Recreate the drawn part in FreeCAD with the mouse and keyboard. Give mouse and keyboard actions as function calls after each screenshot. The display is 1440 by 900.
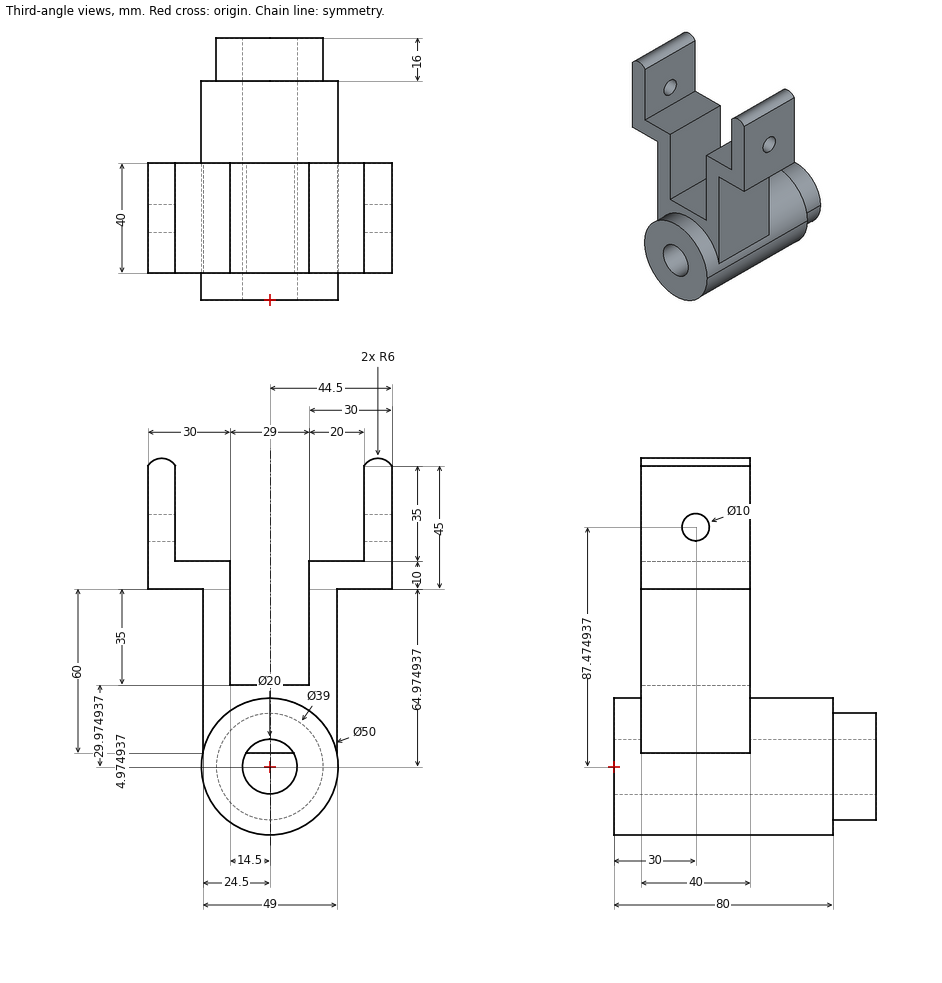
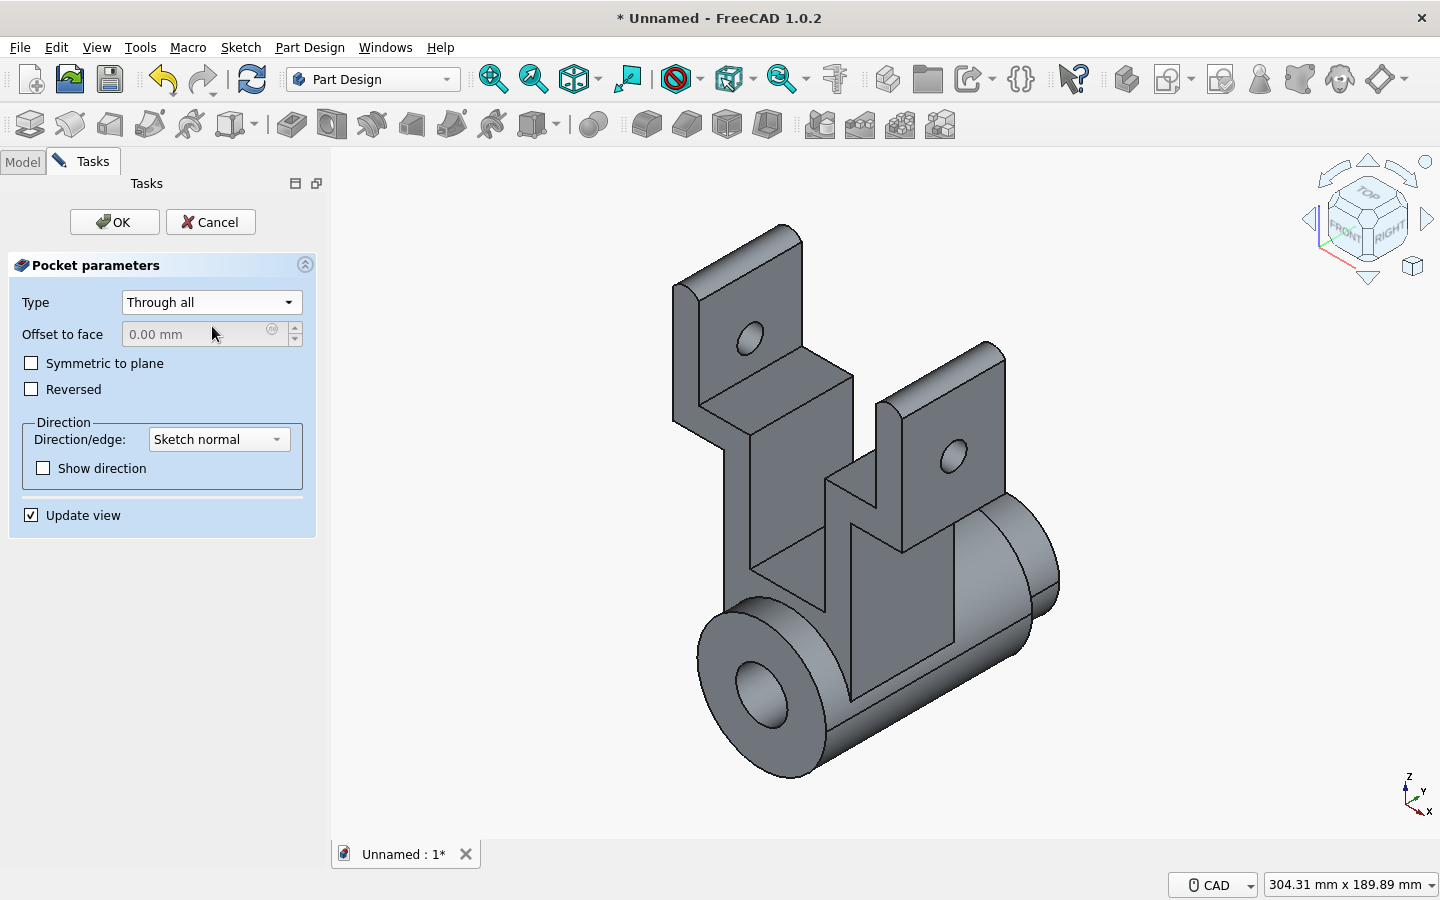
click(115, 222)